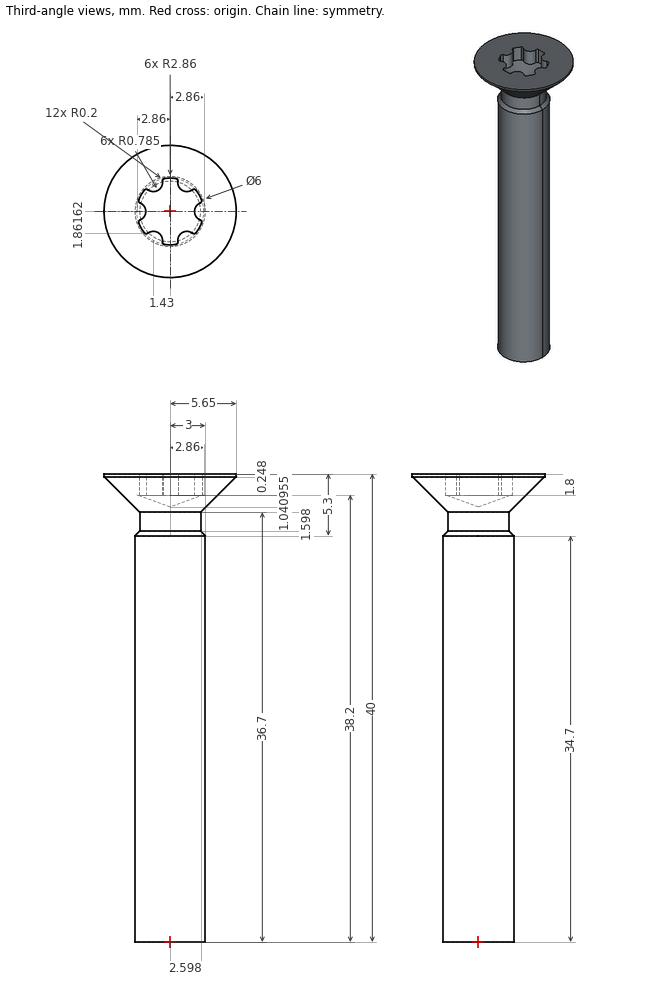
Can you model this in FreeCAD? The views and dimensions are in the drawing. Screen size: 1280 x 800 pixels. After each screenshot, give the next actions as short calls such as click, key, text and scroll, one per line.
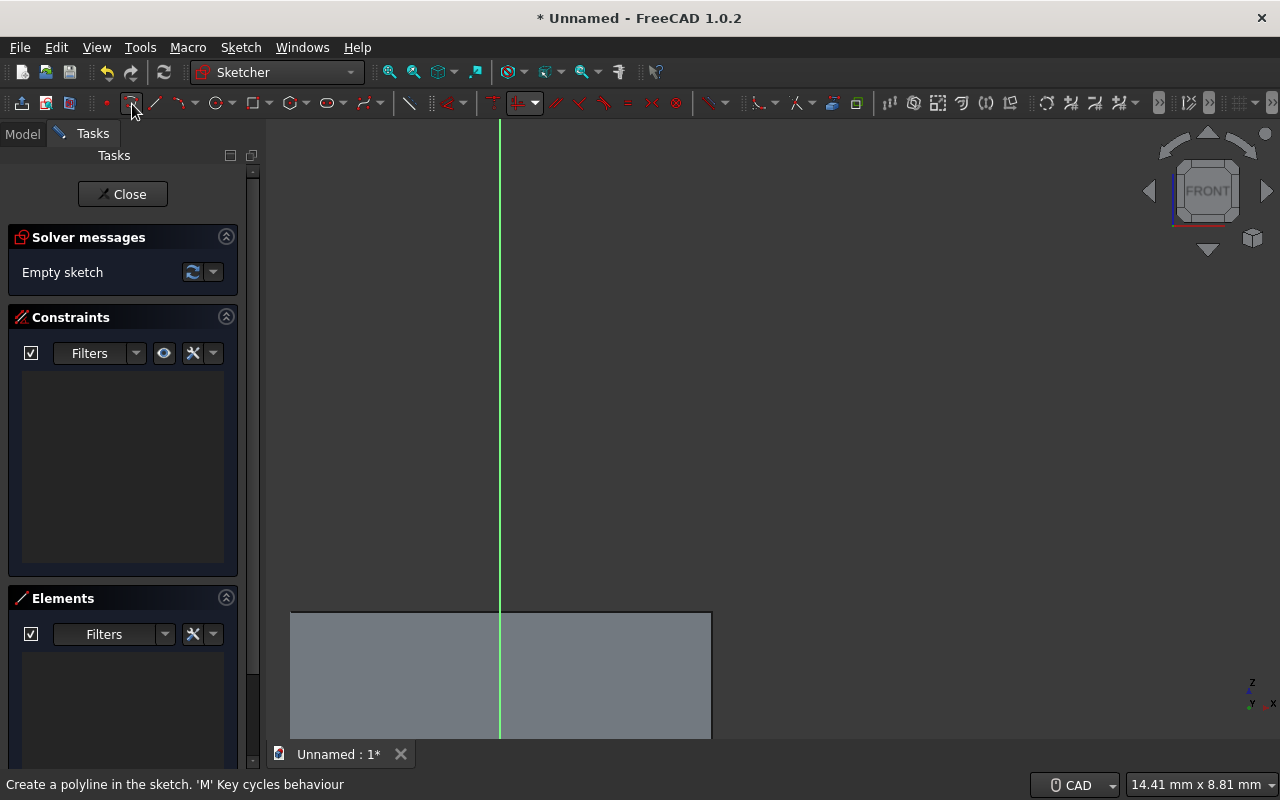
click(500, 612)
click(509, 239)
click(898, 239)
click(898, 256)
click(683, 471)
click(683, 583)
click(712, 612)
click(500, 613)
key(Escape)
key(Escape)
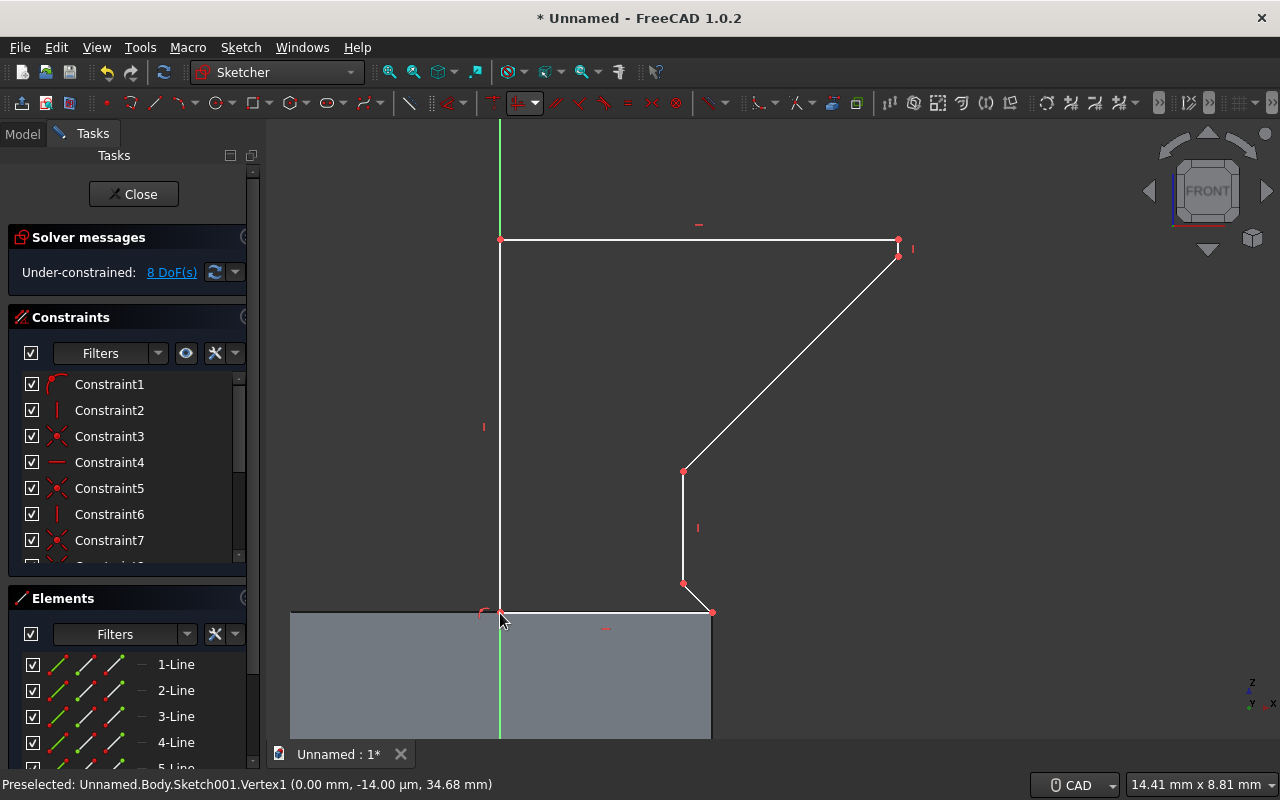
click(649, 613)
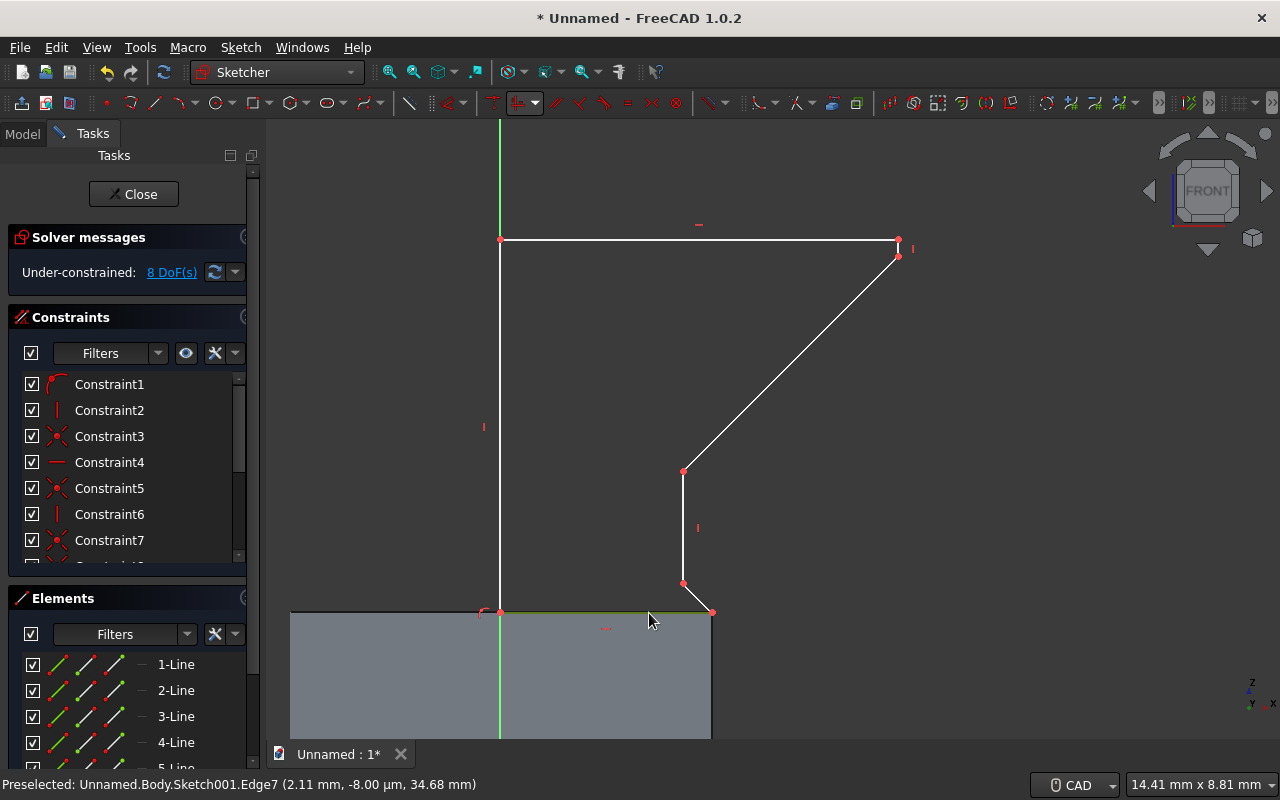
key(l)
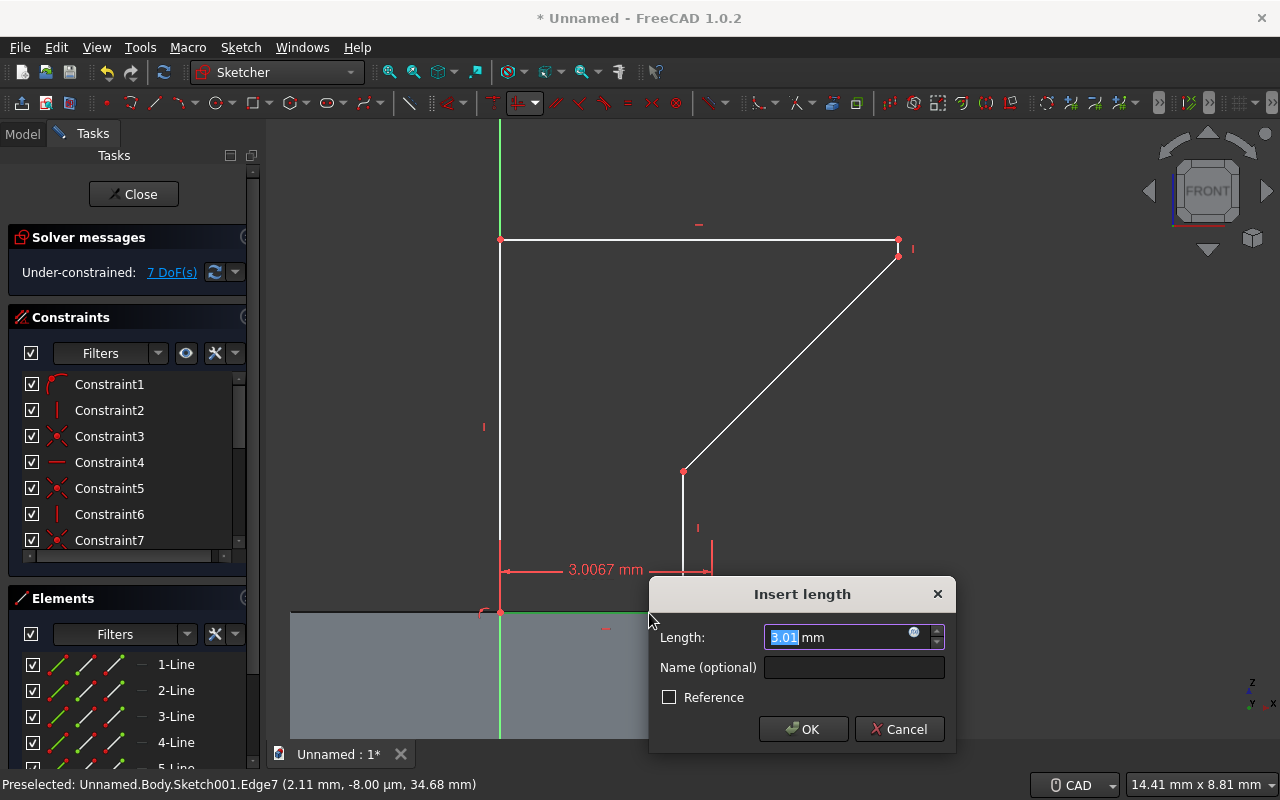
text(3)
key(Return)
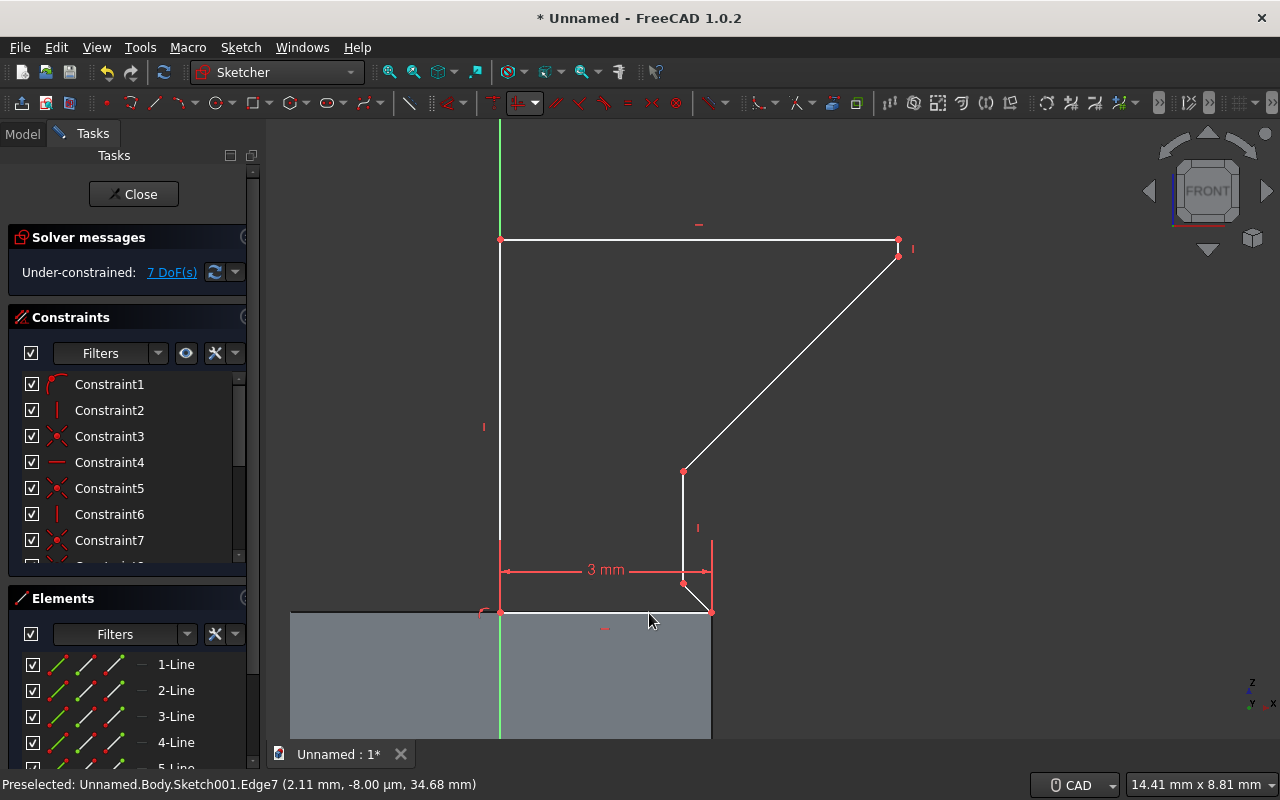
click(500, 501)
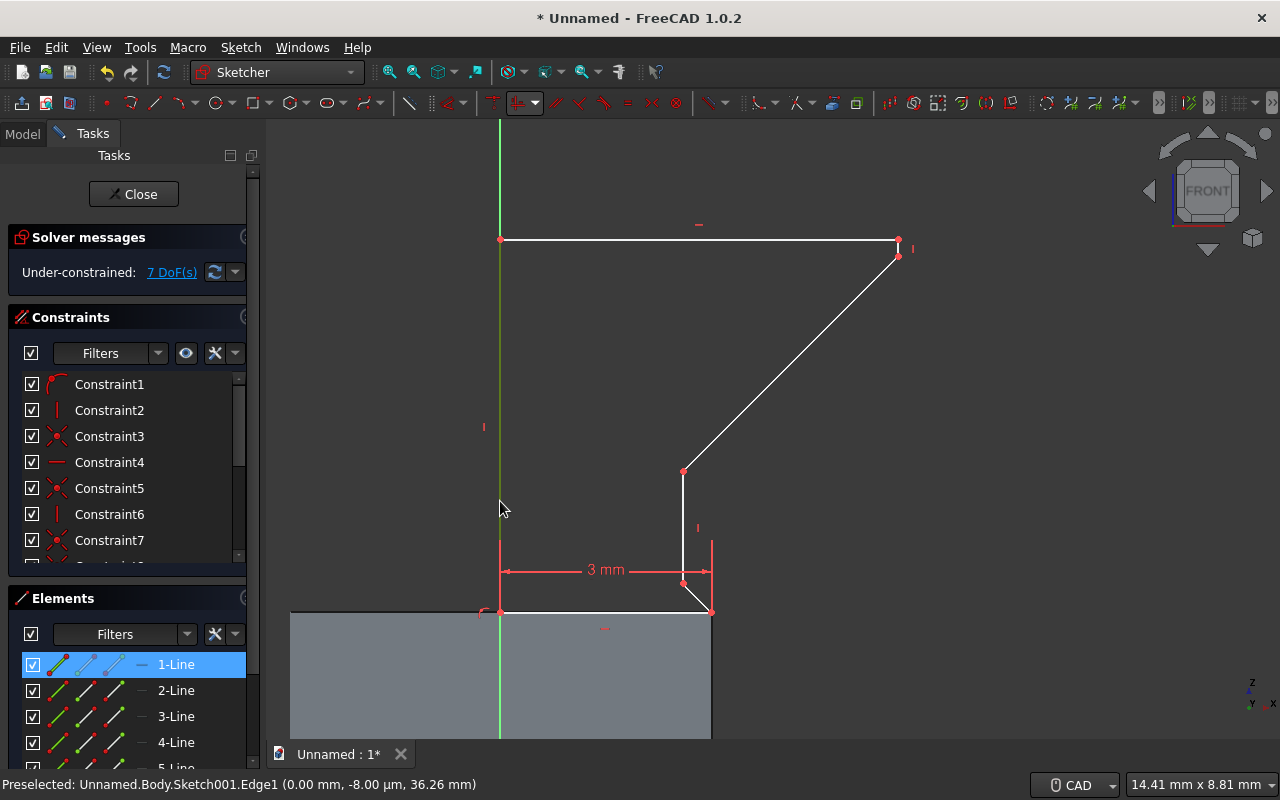
key(i)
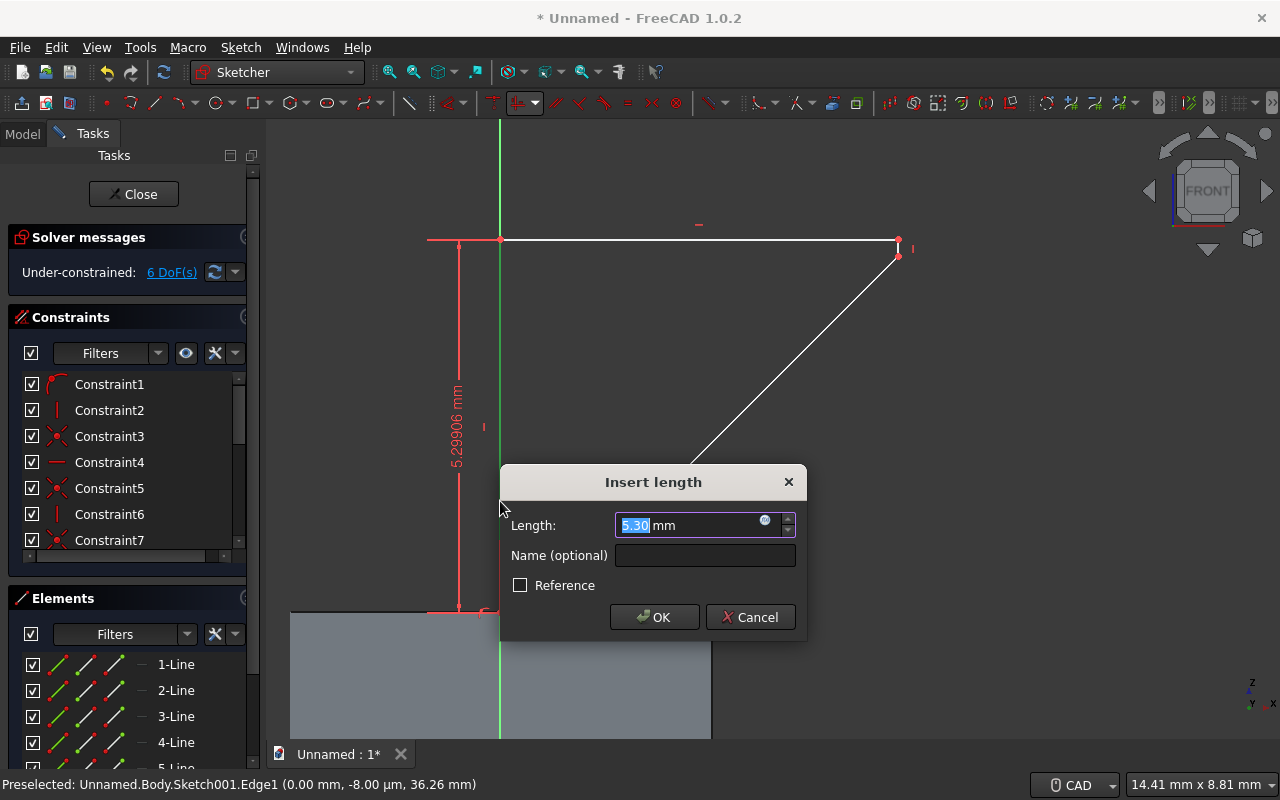
text(5.3)
key(Return)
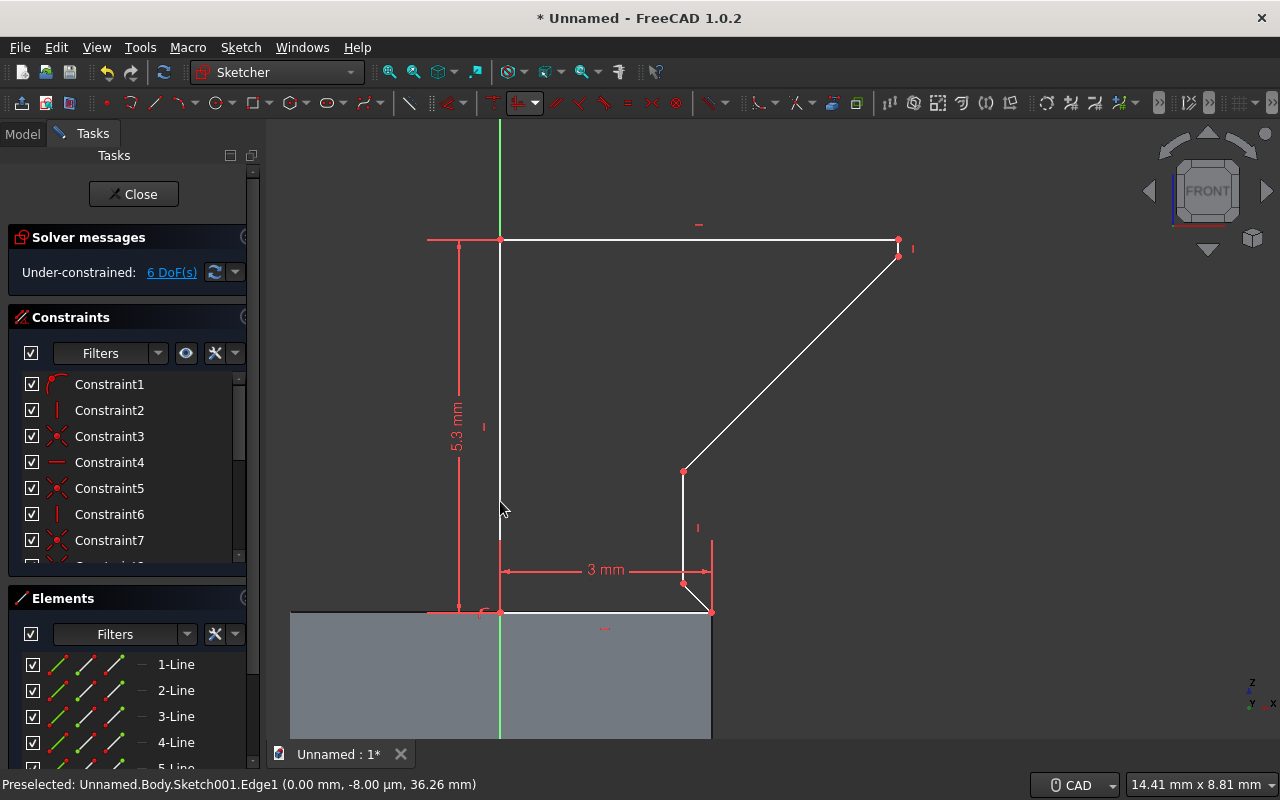
click(500, 240)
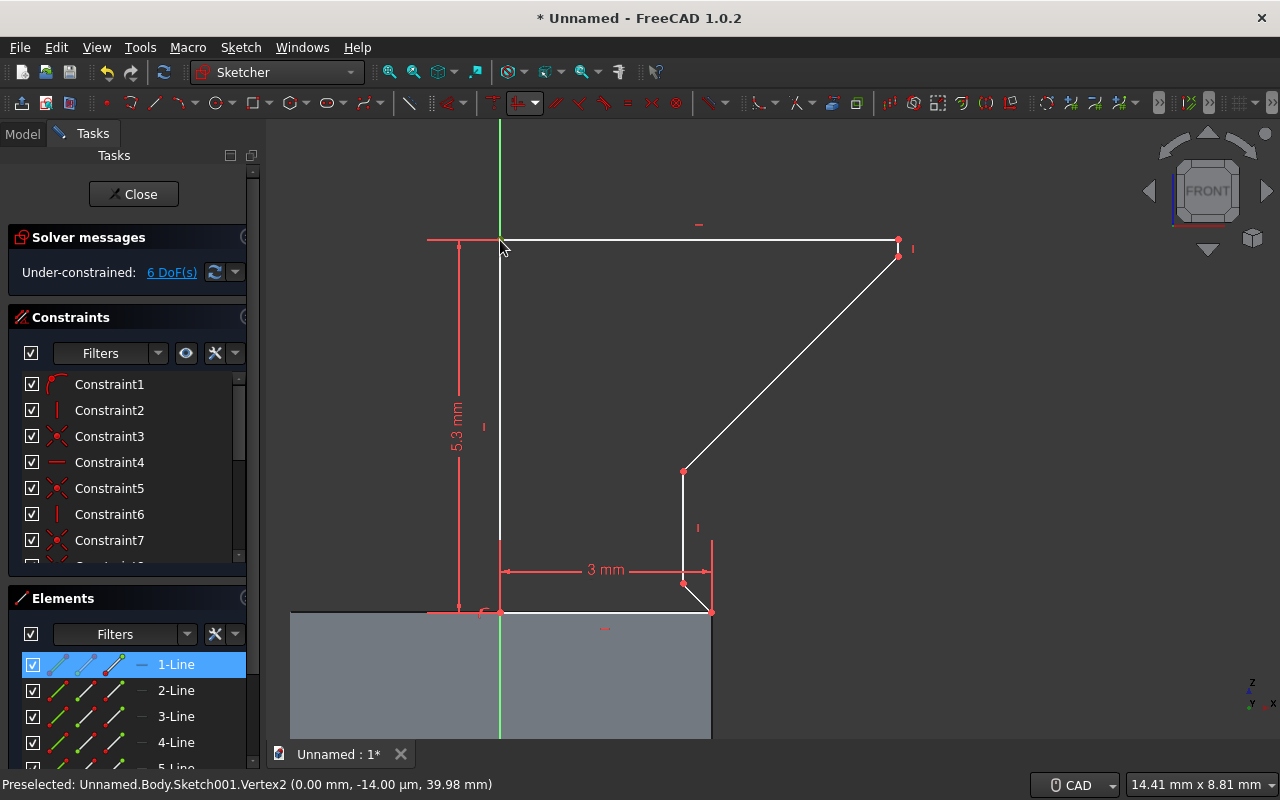
key(i)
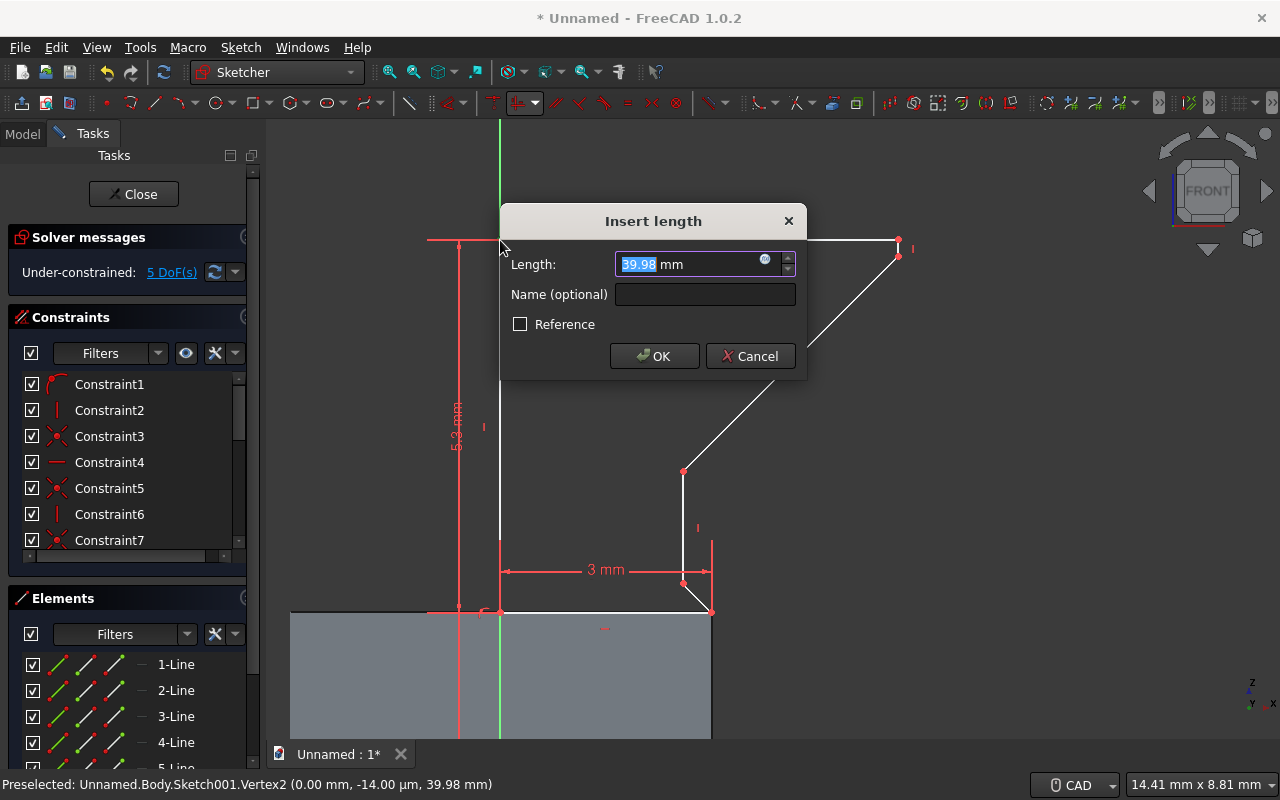
text(40)
key(Return)